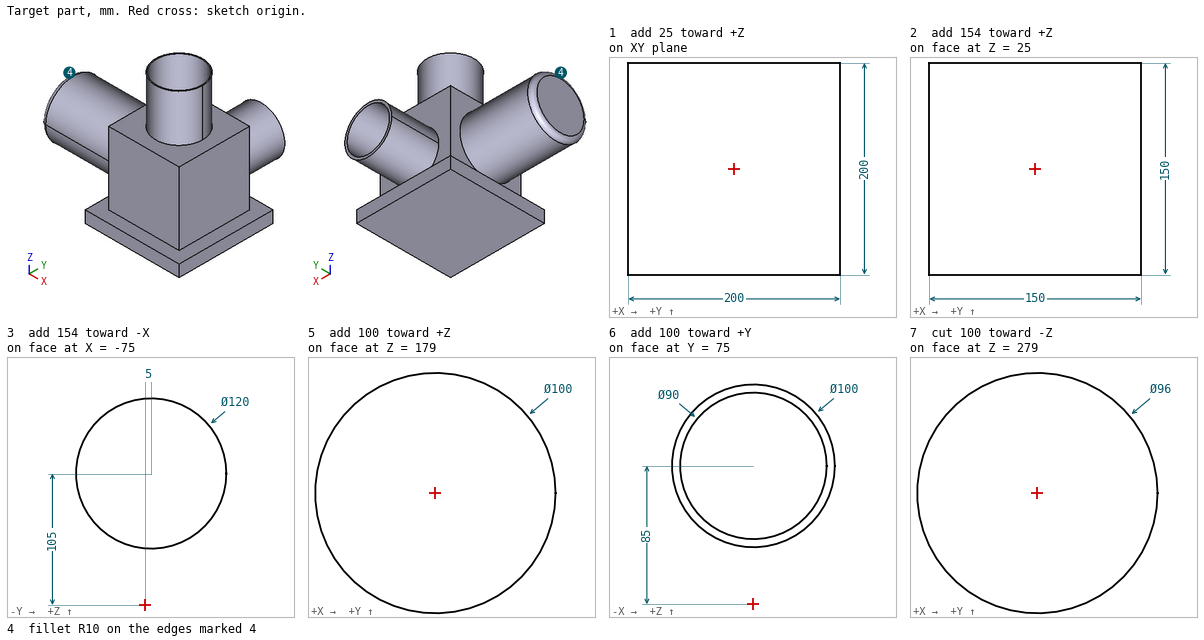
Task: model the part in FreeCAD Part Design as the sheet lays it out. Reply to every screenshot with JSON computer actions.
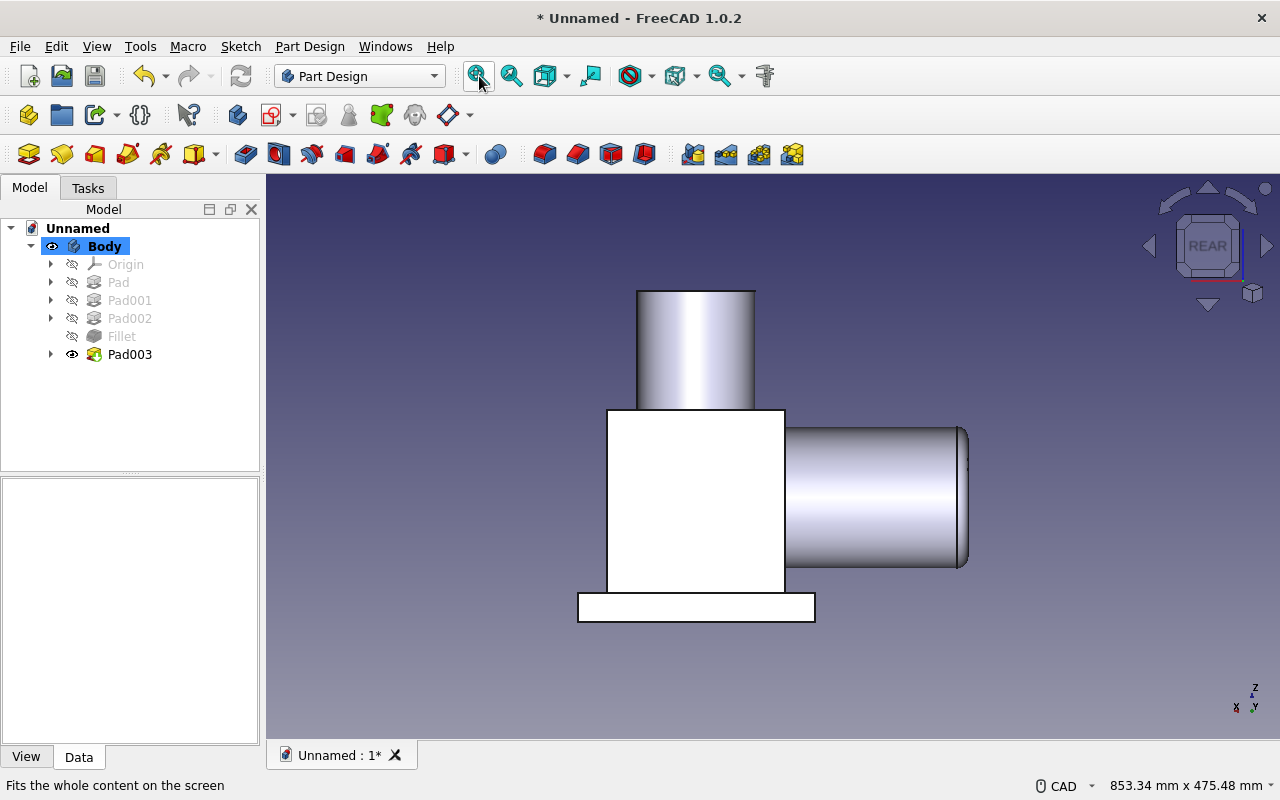
{"action": "left_click", "coordinate": [696, 500]}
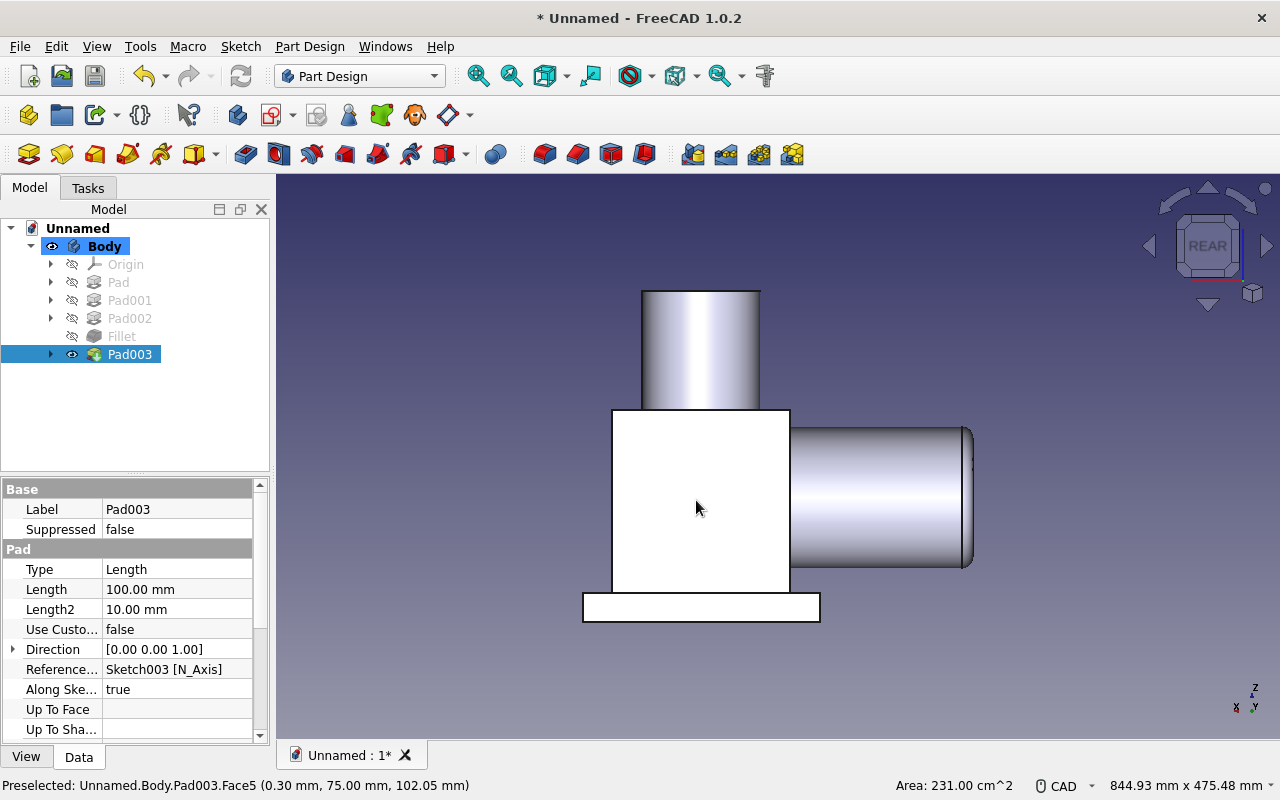
{"action": "left_click", "coordinate": [270, 116]}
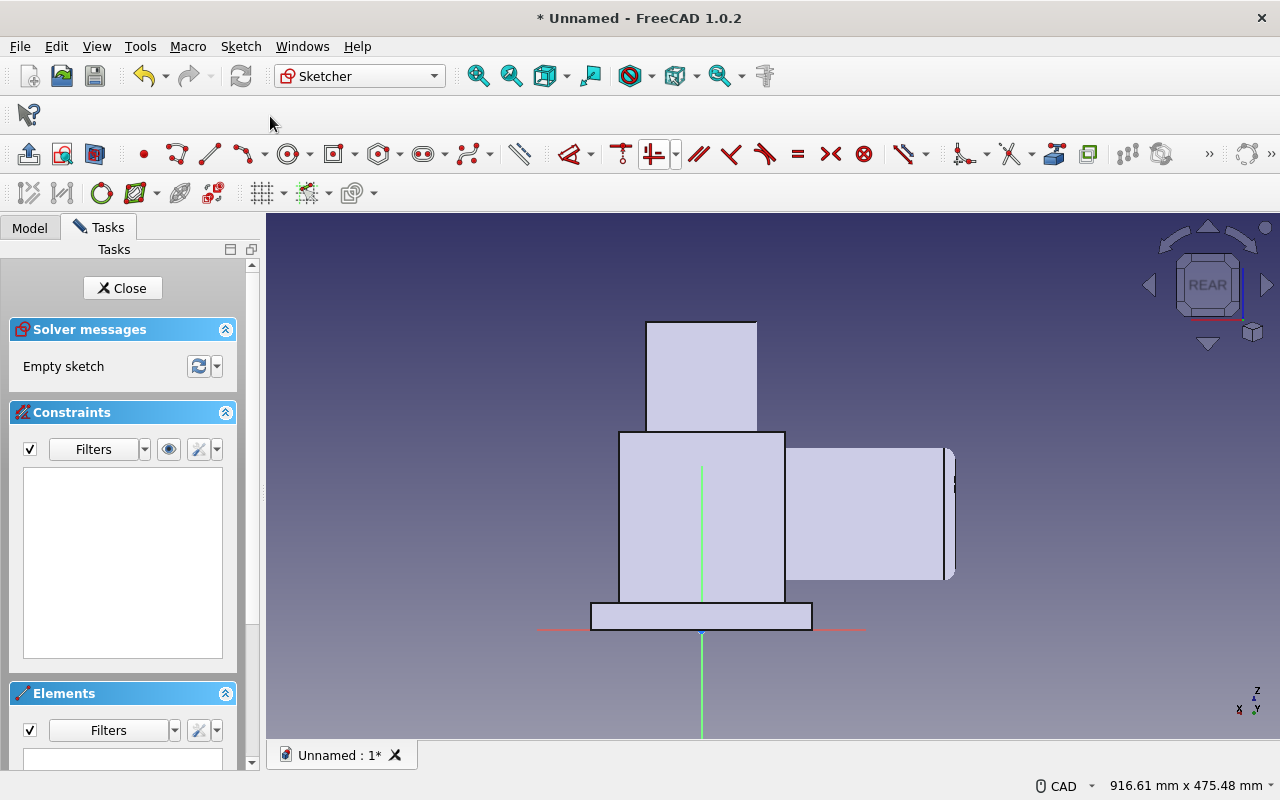
{"action": "left_click", "coordinate": [95, 154]}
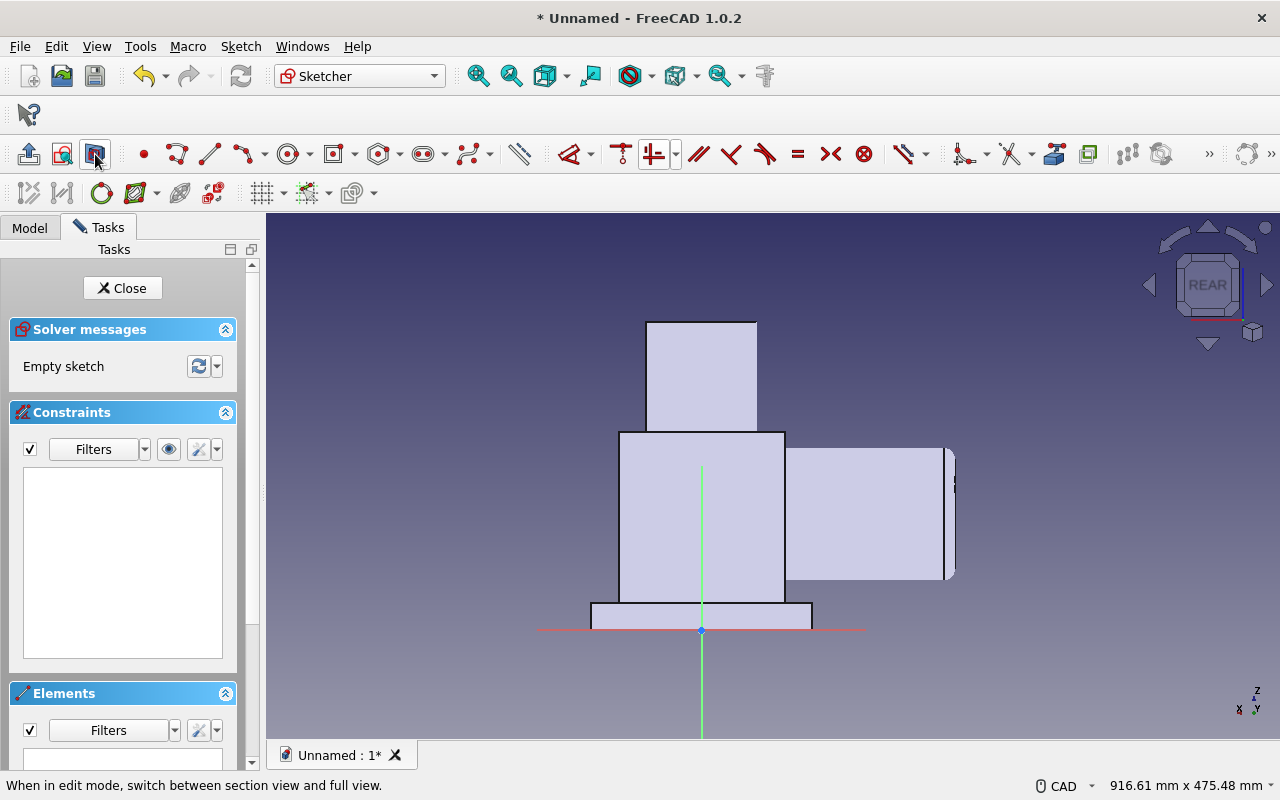
{"action": "scroll", "coordinate": [699, 621], "scroll_direction": "up", "scroll_amount": 4}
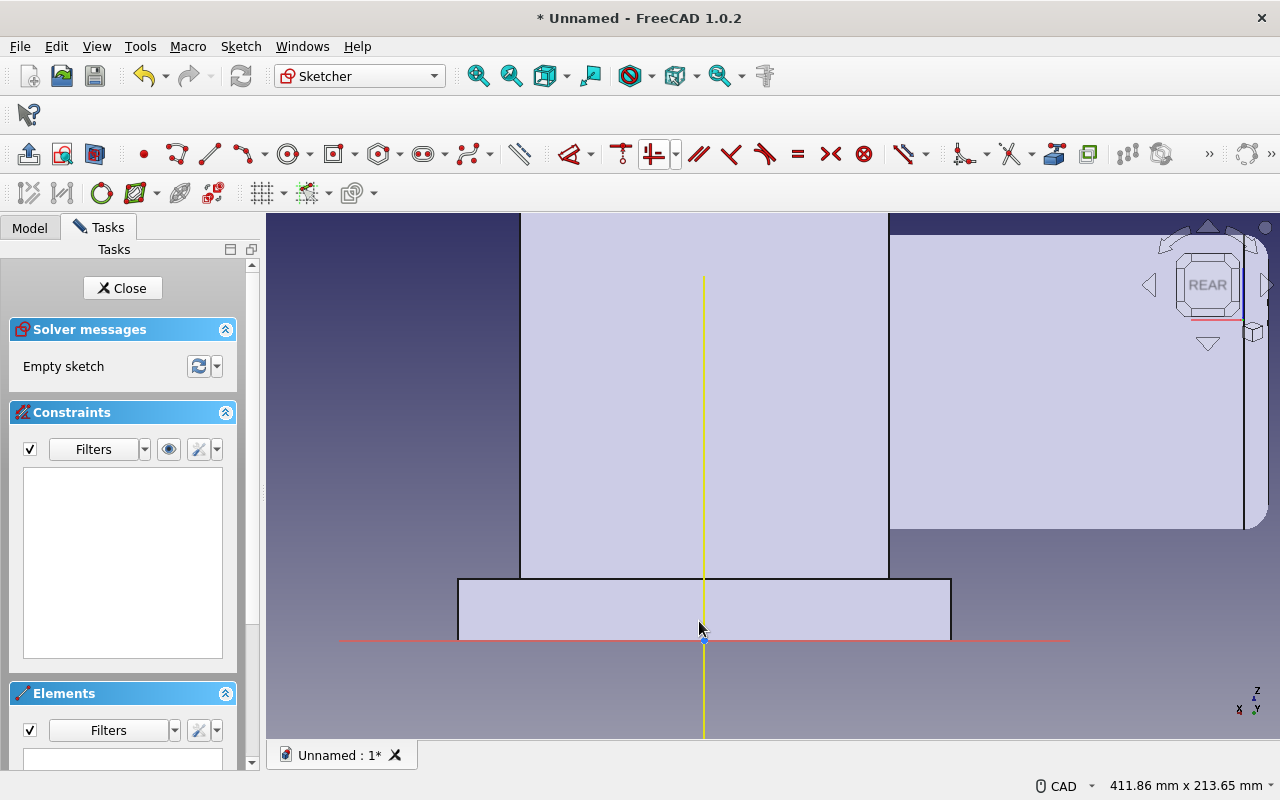
{"action": "left_click", "coordinate": [288, 154]}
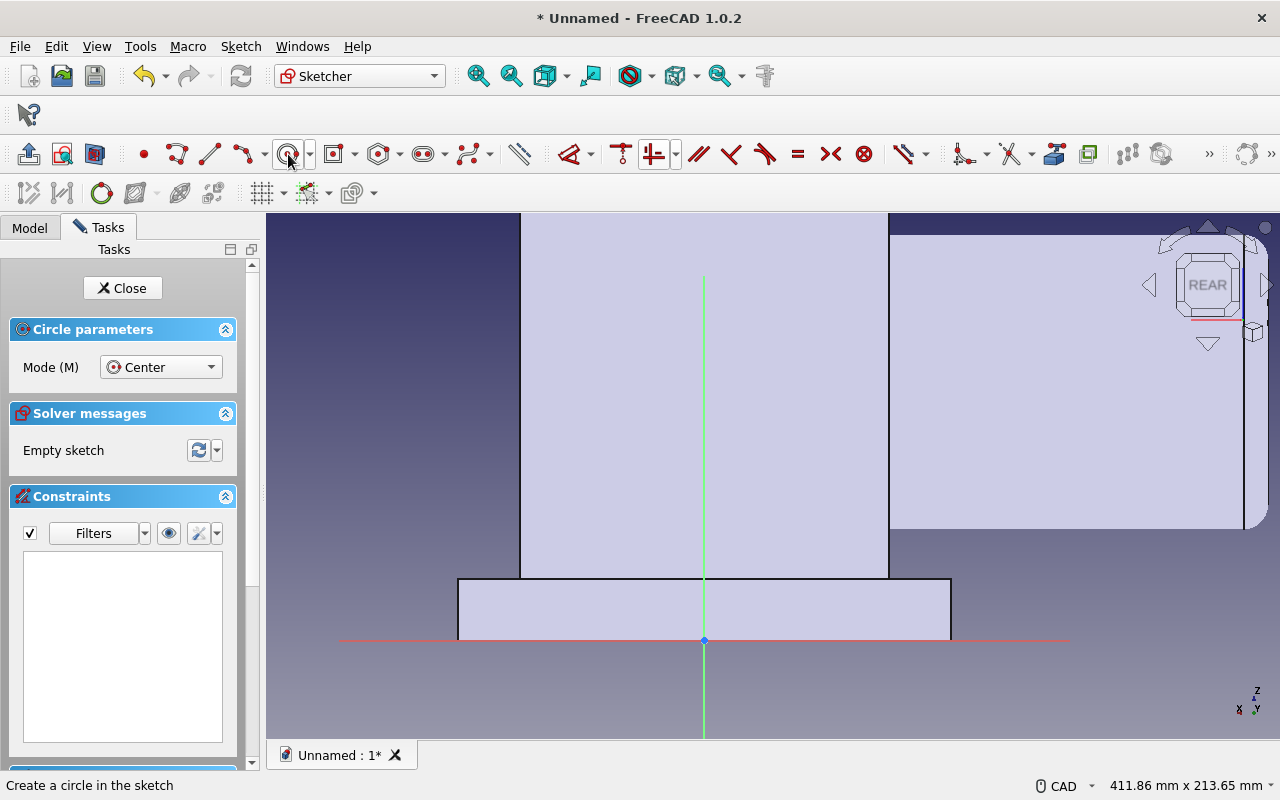
{"action": "left_click", "coordinate": [704, 432]}
{"action": "mouse_move", "coordinate": [791, 344]}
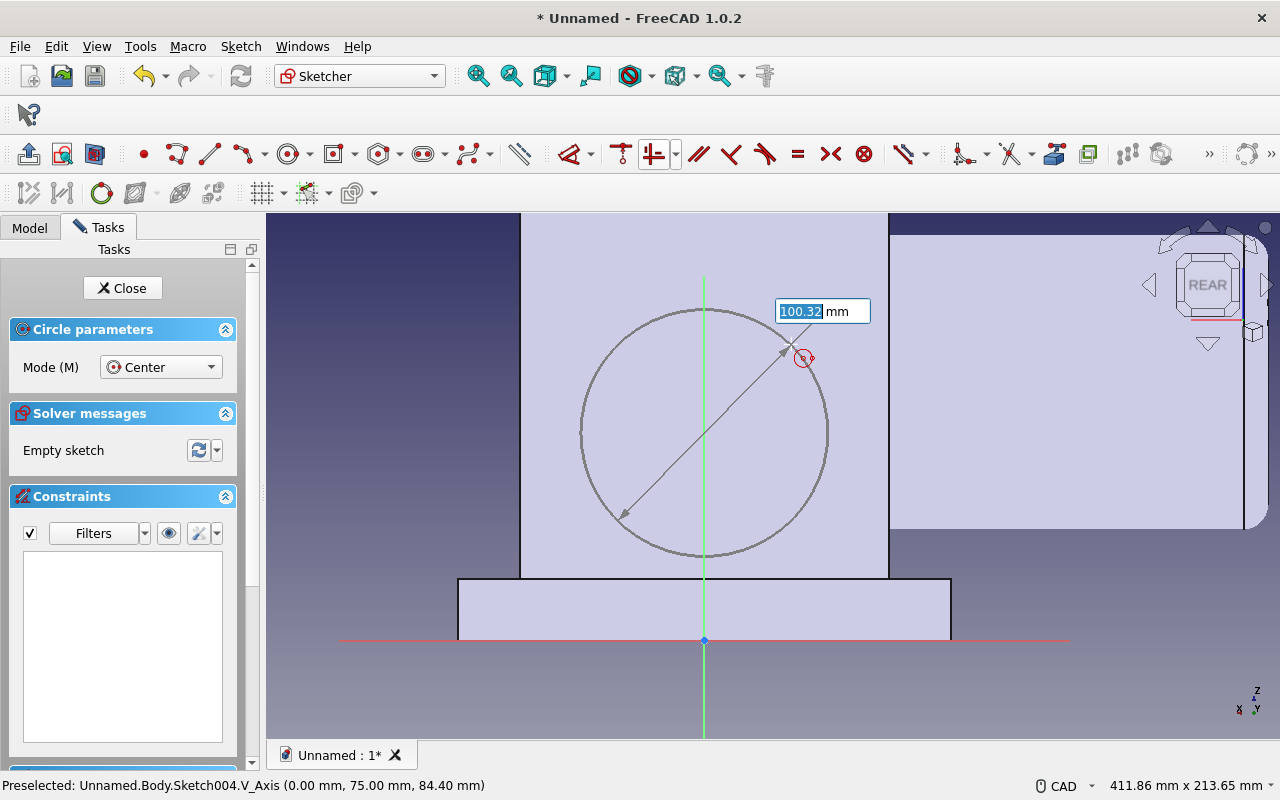
{"action": "type", "text": "100"}
{"action": "key", "text": "Return"}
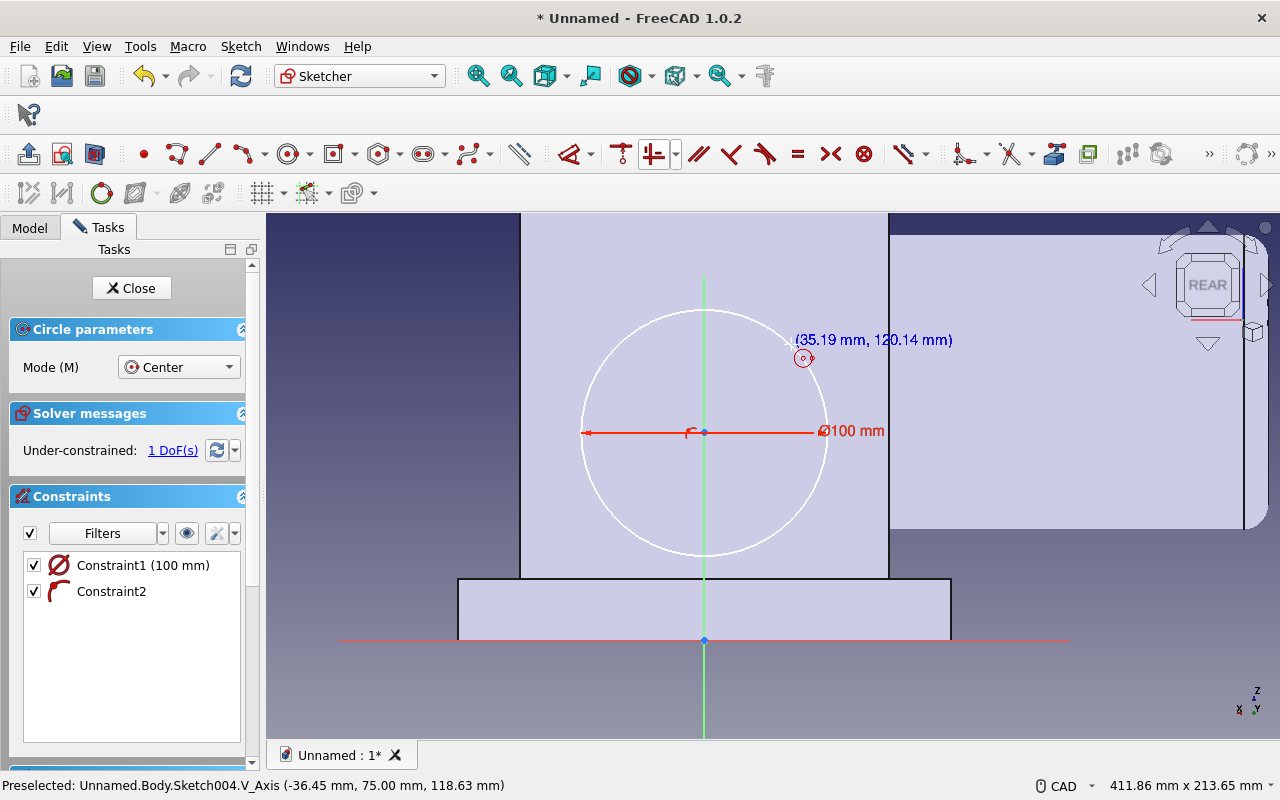
{"action": "left_click", "coordinate": [704, 433]}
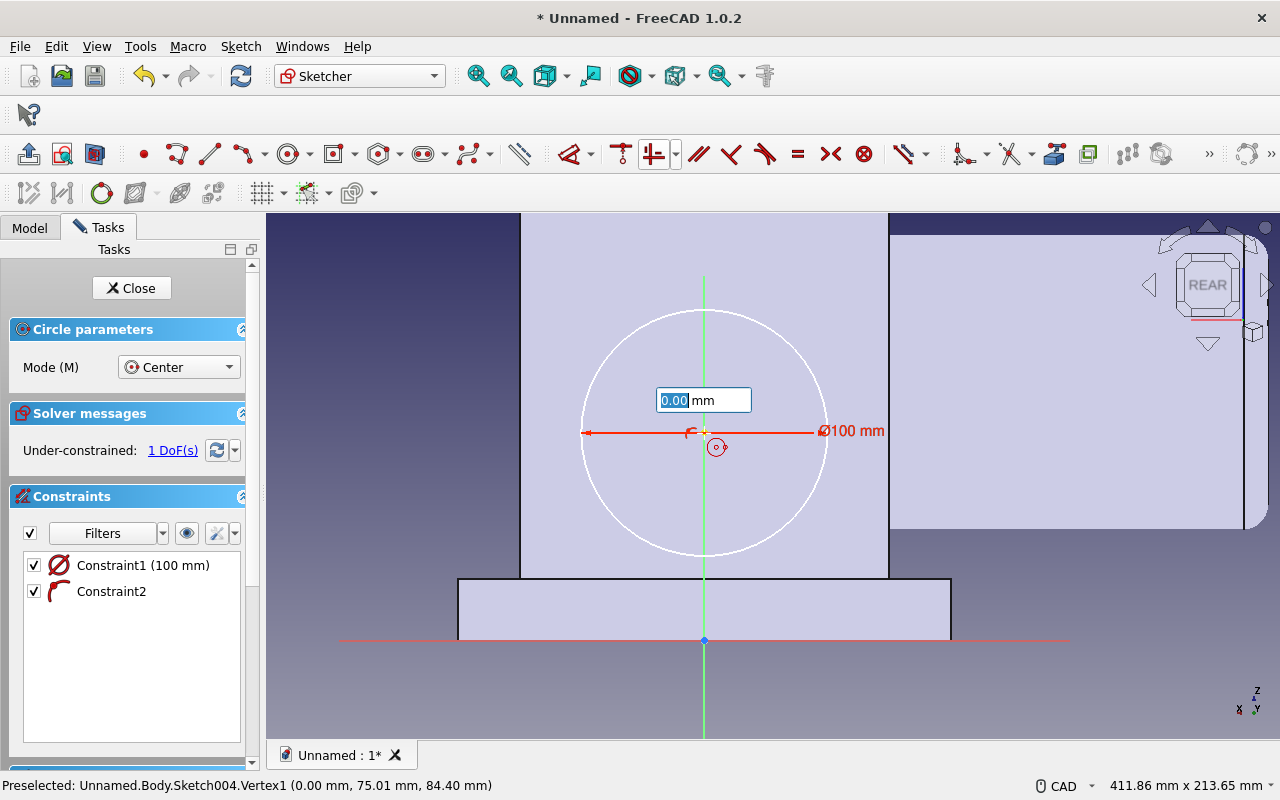
{"action": "scroll", "coordinate": [783, 353], "scroll_direction": "up", "scroll_amount": 2}
{"action": "mouse_move", "coordinate": [782, 353]}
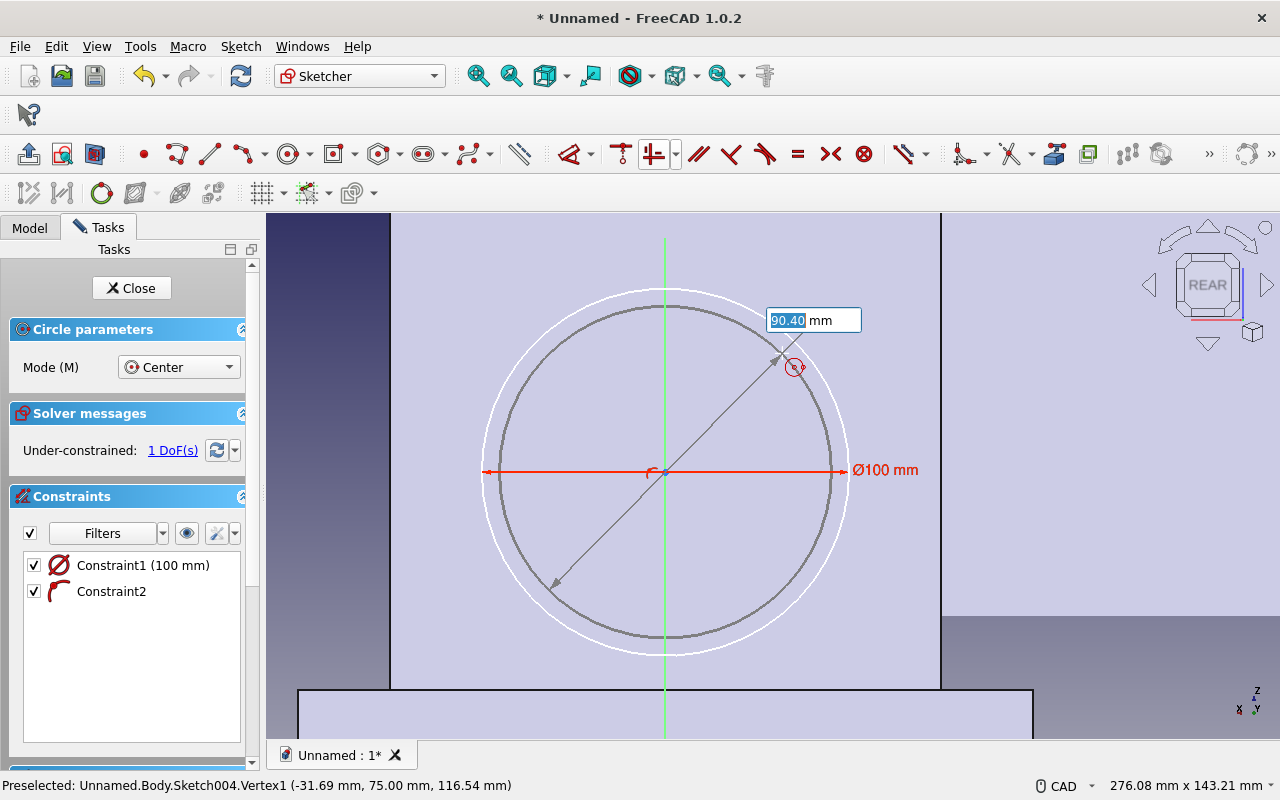
{"action": "type", "text": "90"}
{"action": "key", "text": "Return"}
{"action": "key", "text": "Escape"}